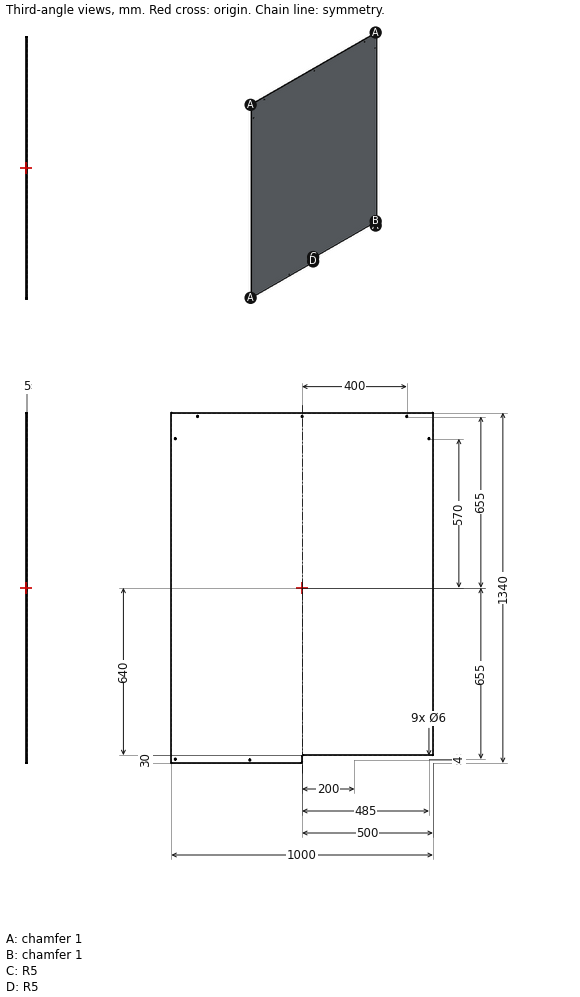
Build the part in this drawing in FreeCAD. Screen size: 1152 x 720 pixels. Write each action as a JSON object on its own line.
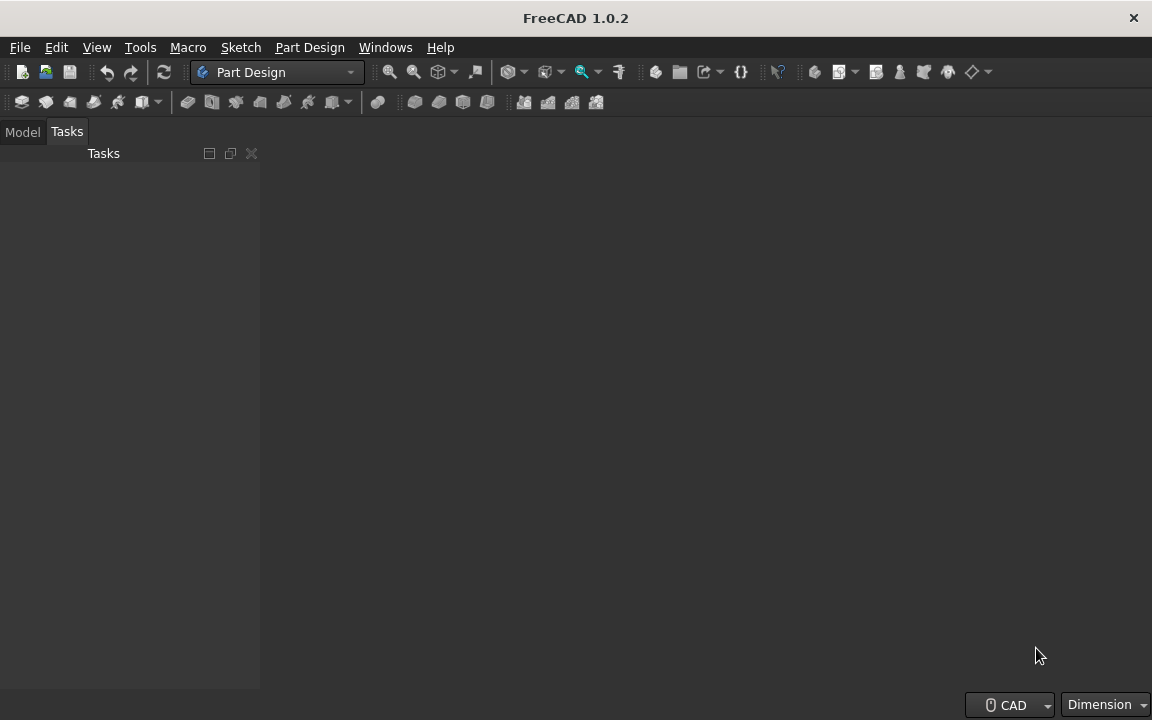
{"action": "left_click", "coordinate": [22, 72]}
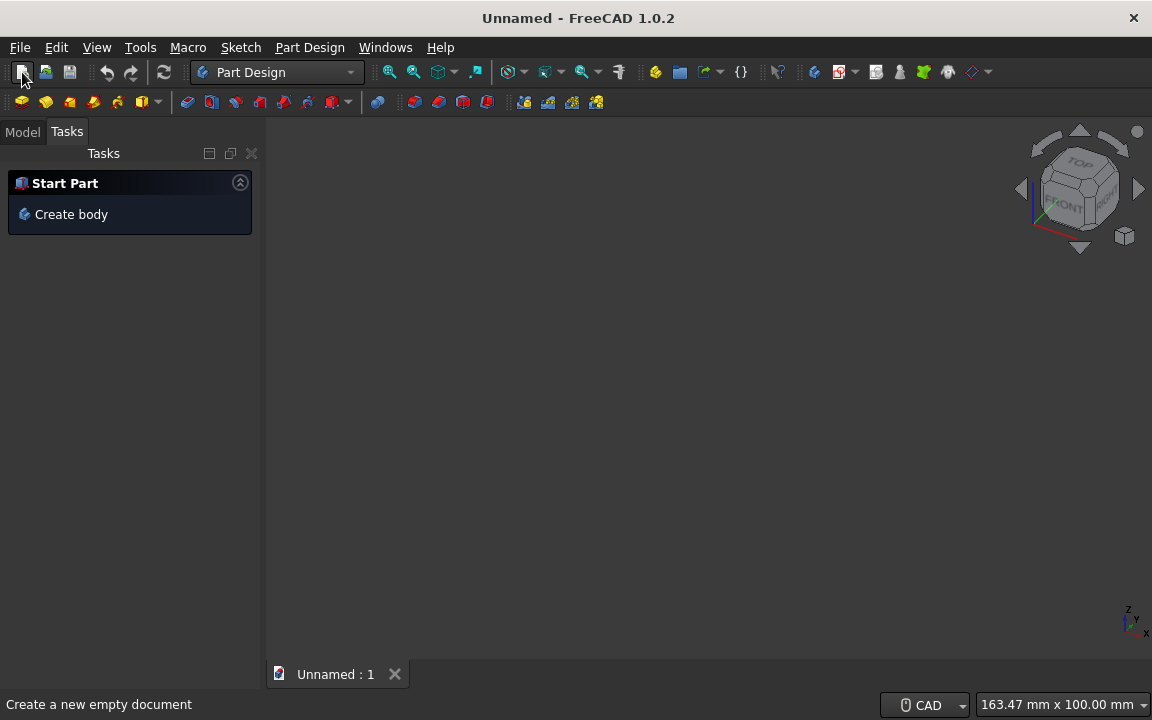
{"action": "left_click", "coordinate": [840, 72]}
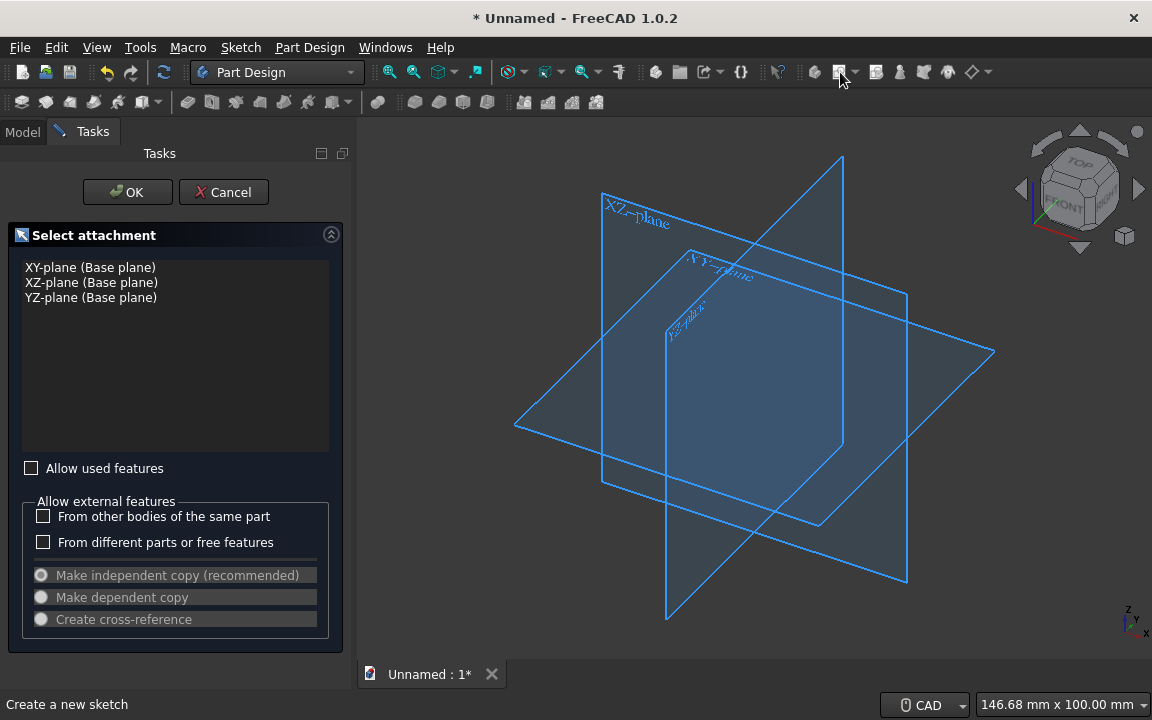
{"action": "left_click", "coordinate": [82, 298]}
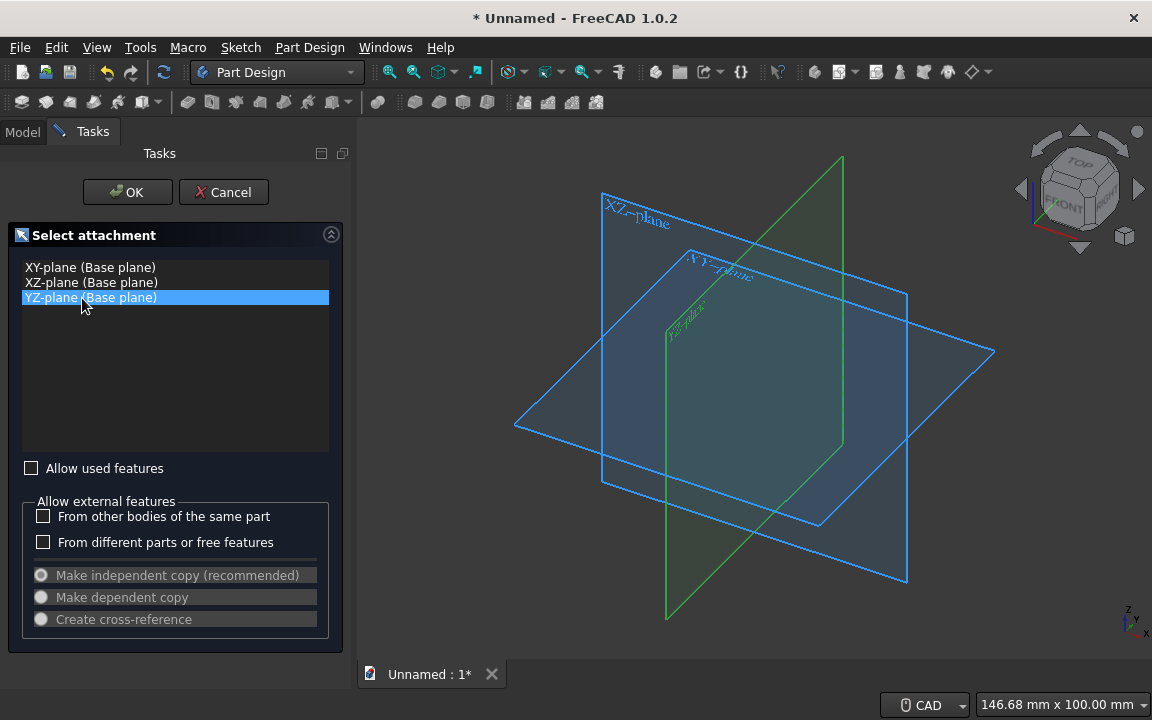
{"action": "left_click", "coordinate": [128, 192]}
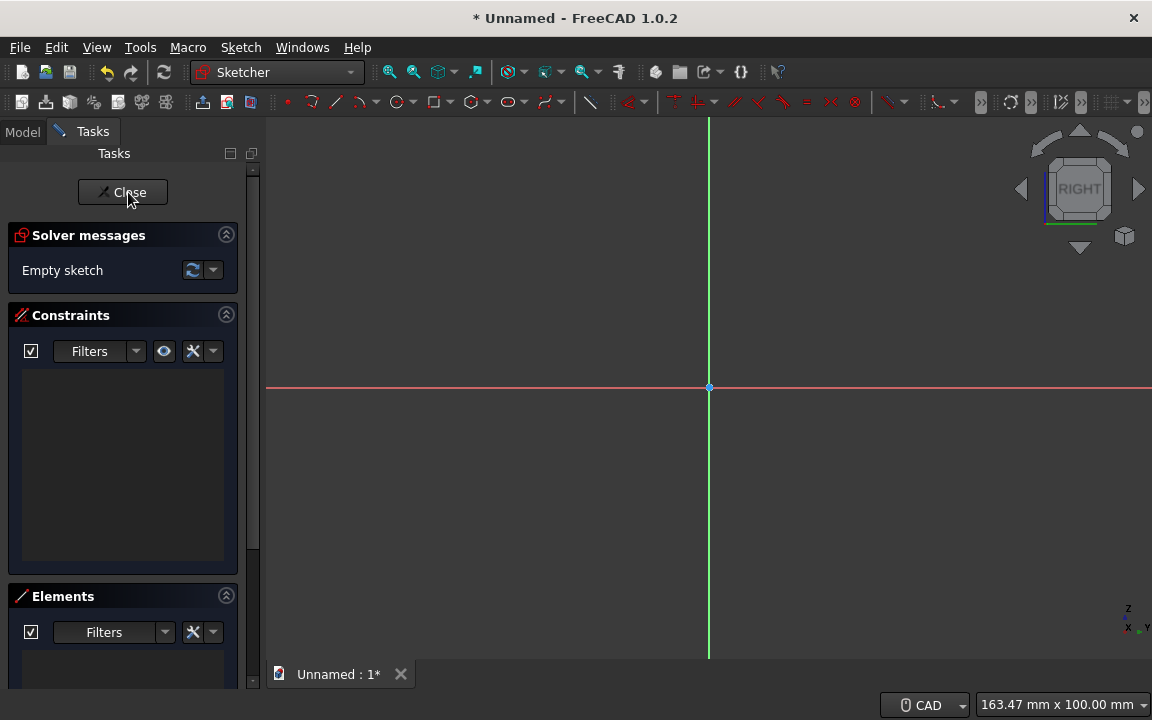
{"action": "scroll", "coordinate": [637, 388], "scroll_direction": "down", "scroll_amount": 15}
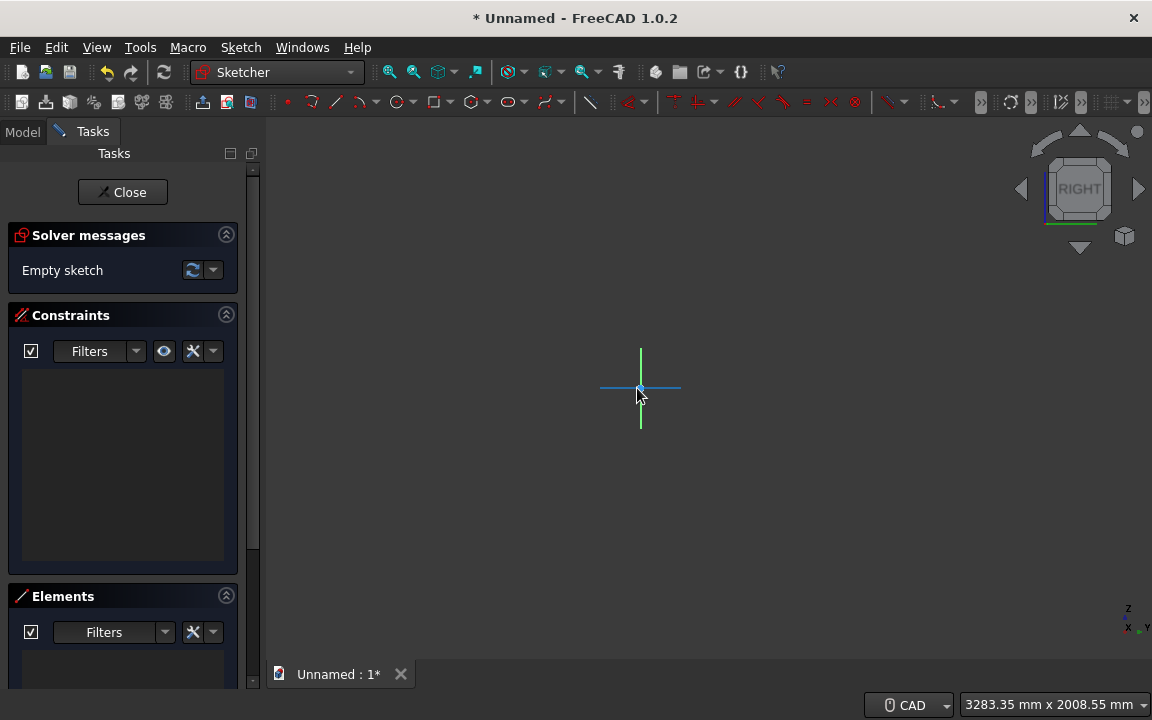
{"action": "left_click", "coordinate": [452, 102]}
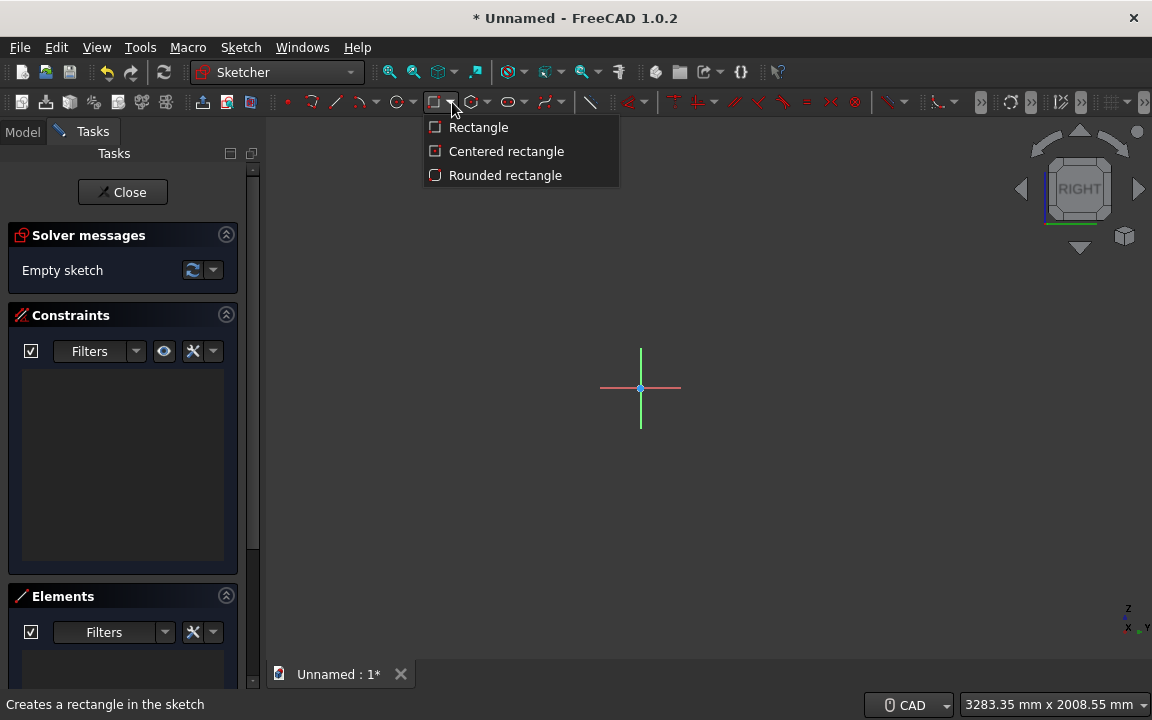
{"action": "left_click", "coordinate": [522, 151]}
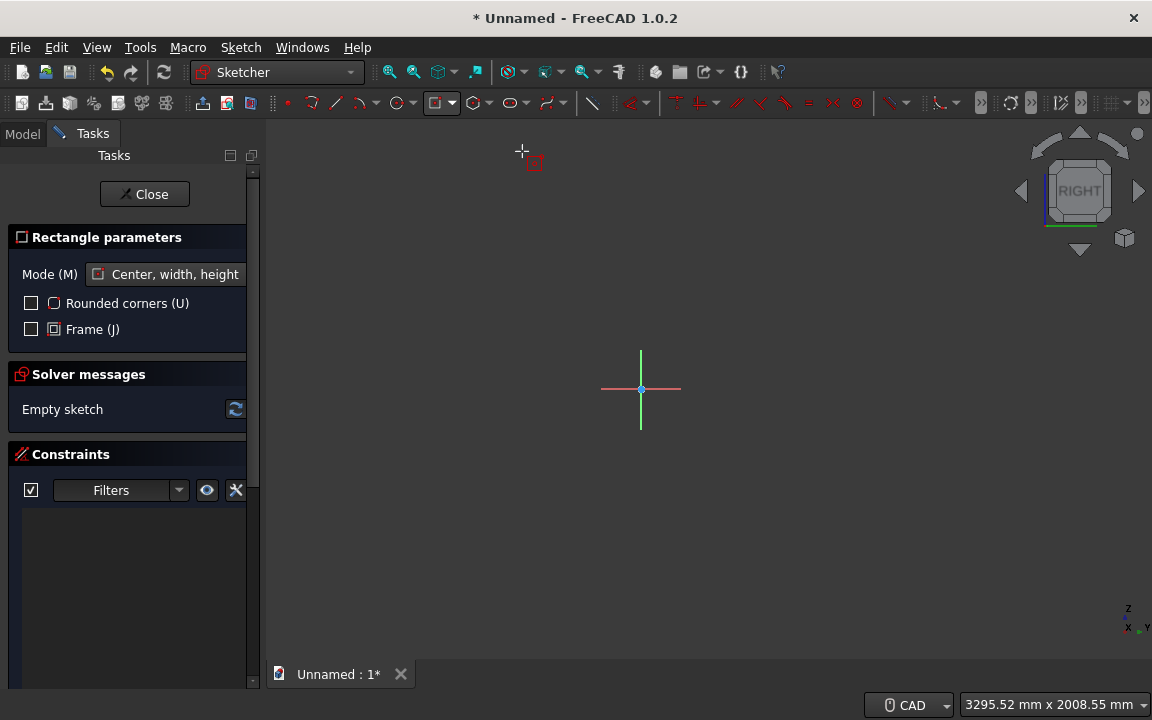
{"action": "left_click", "coordinate": [641, 389]}
{"action": "left_click", "coordinate": [776, 209]}
{"action": "key", "text": "Escape"}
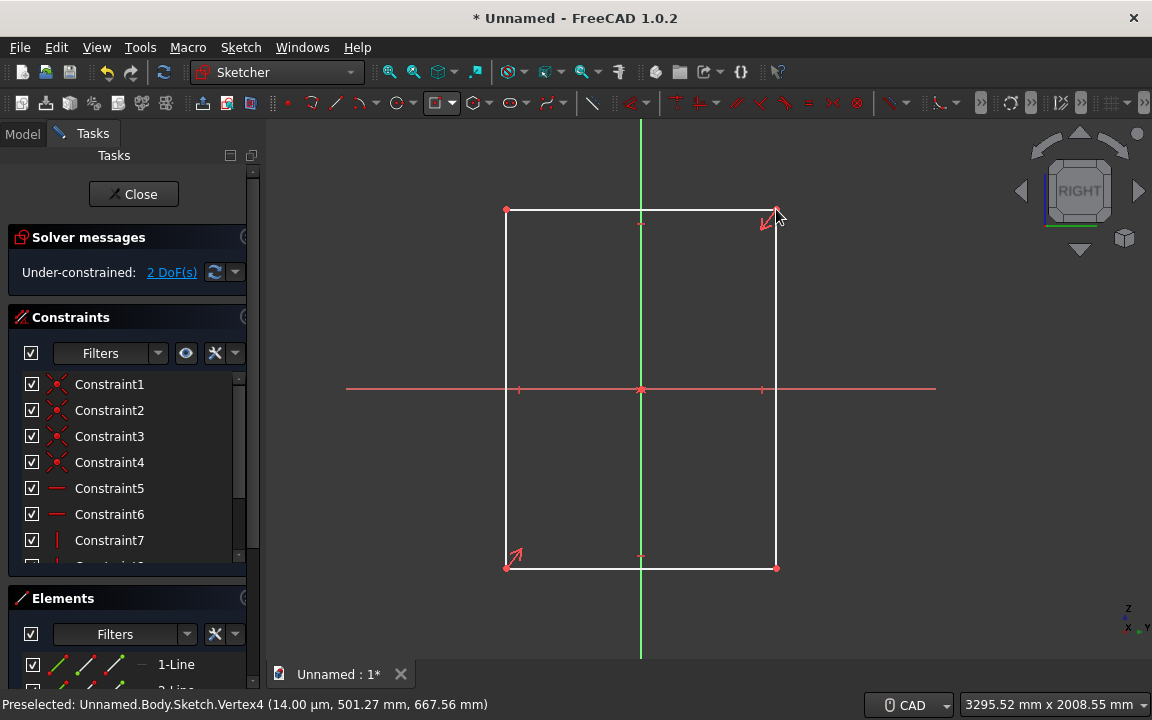
{"action": "left_click", "coordinate": [630, 104]}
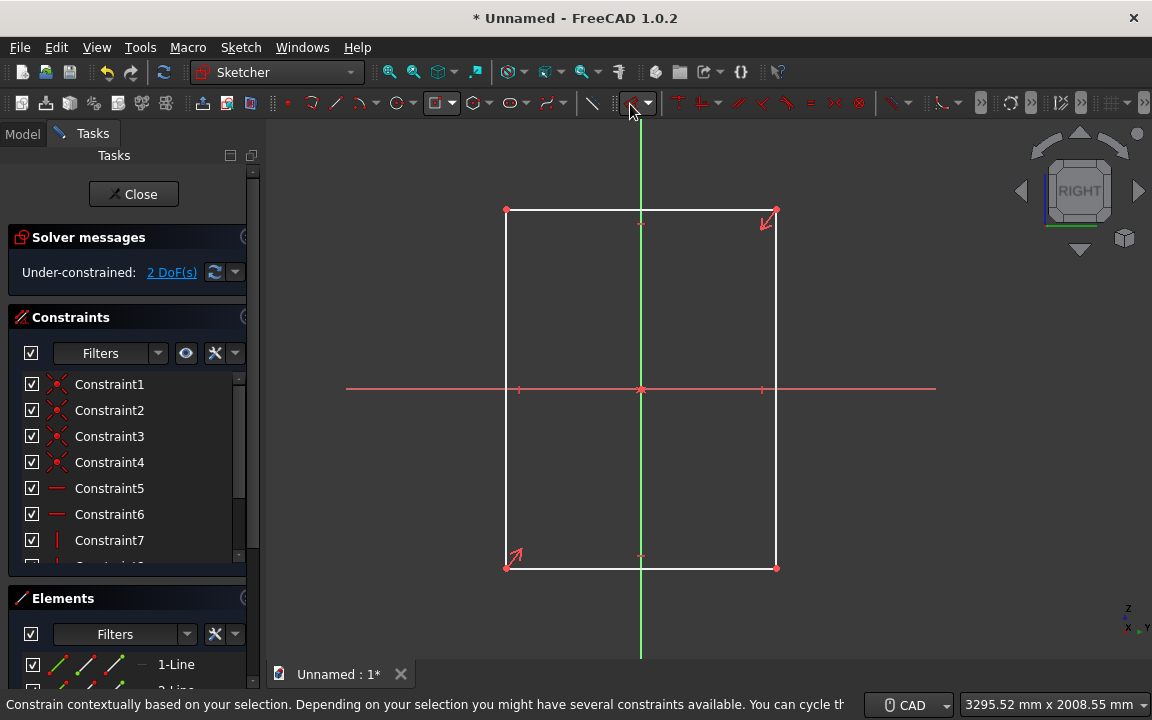
{"action": "left_click", "coordinate": [587, 569]}
{"action": "left_click", "coordinate": [579, 603]}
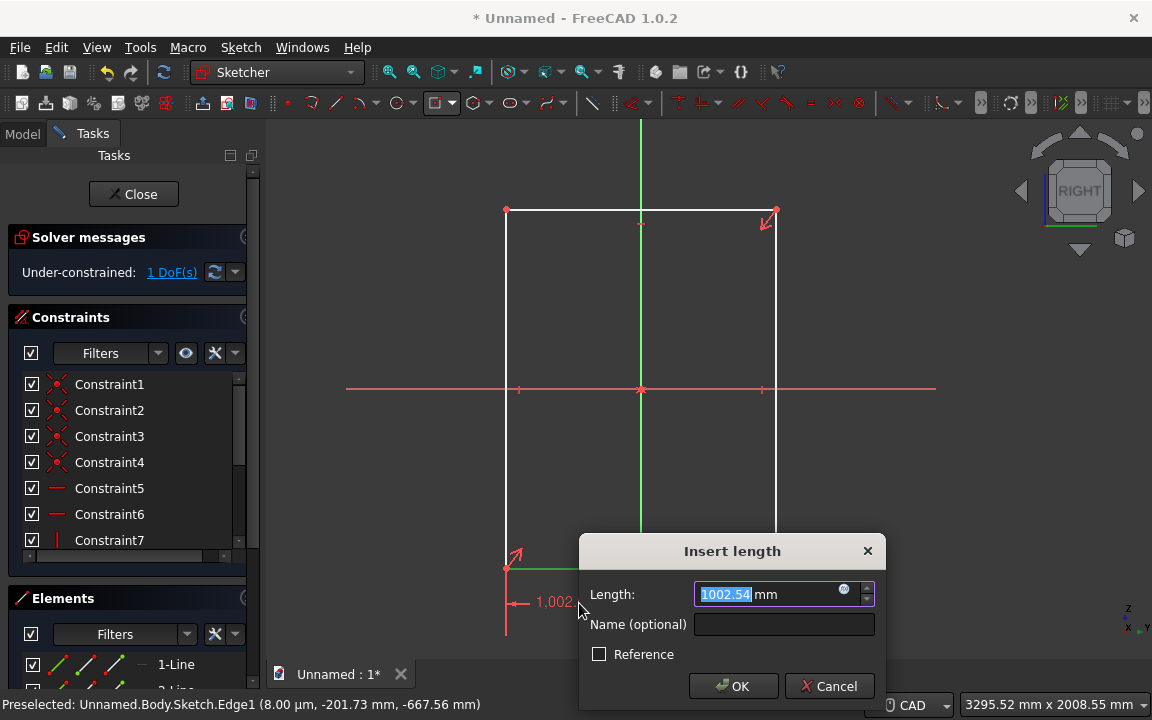
{"action": "type", "text": "1000"}
{"action": "key", "text": "Return"}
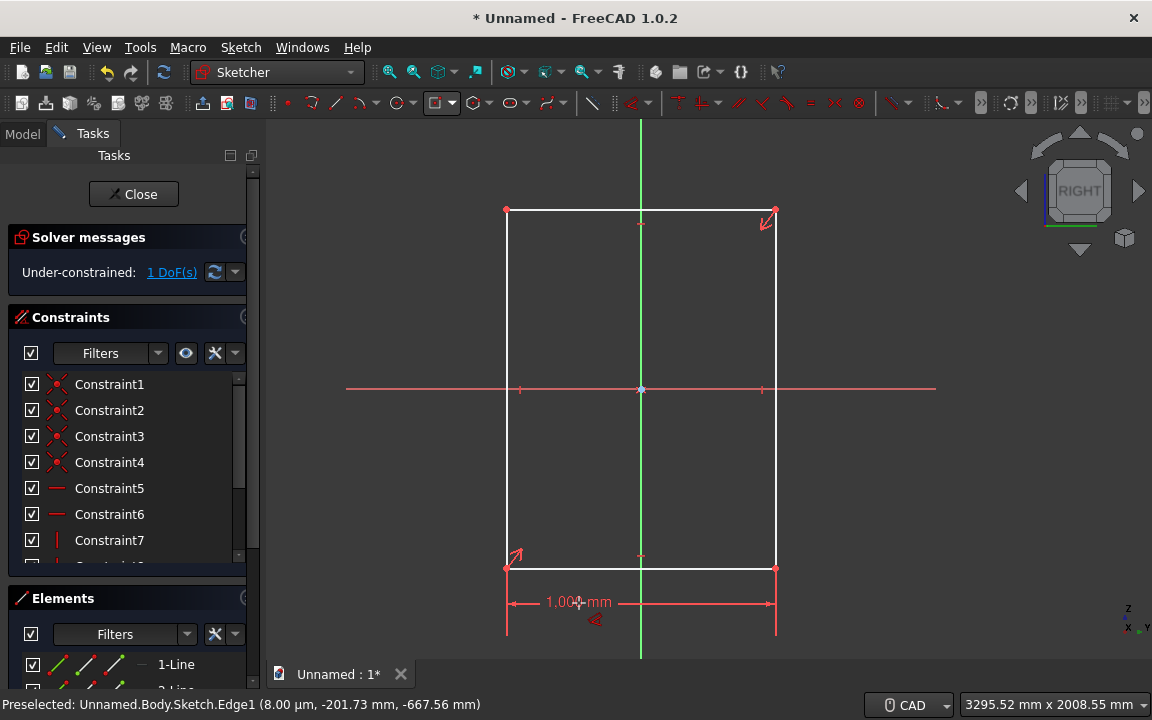
{"action": "left_click", "coordinate": [776, 461]}
{"action": "left_click", "coordinate": [810, 307]}